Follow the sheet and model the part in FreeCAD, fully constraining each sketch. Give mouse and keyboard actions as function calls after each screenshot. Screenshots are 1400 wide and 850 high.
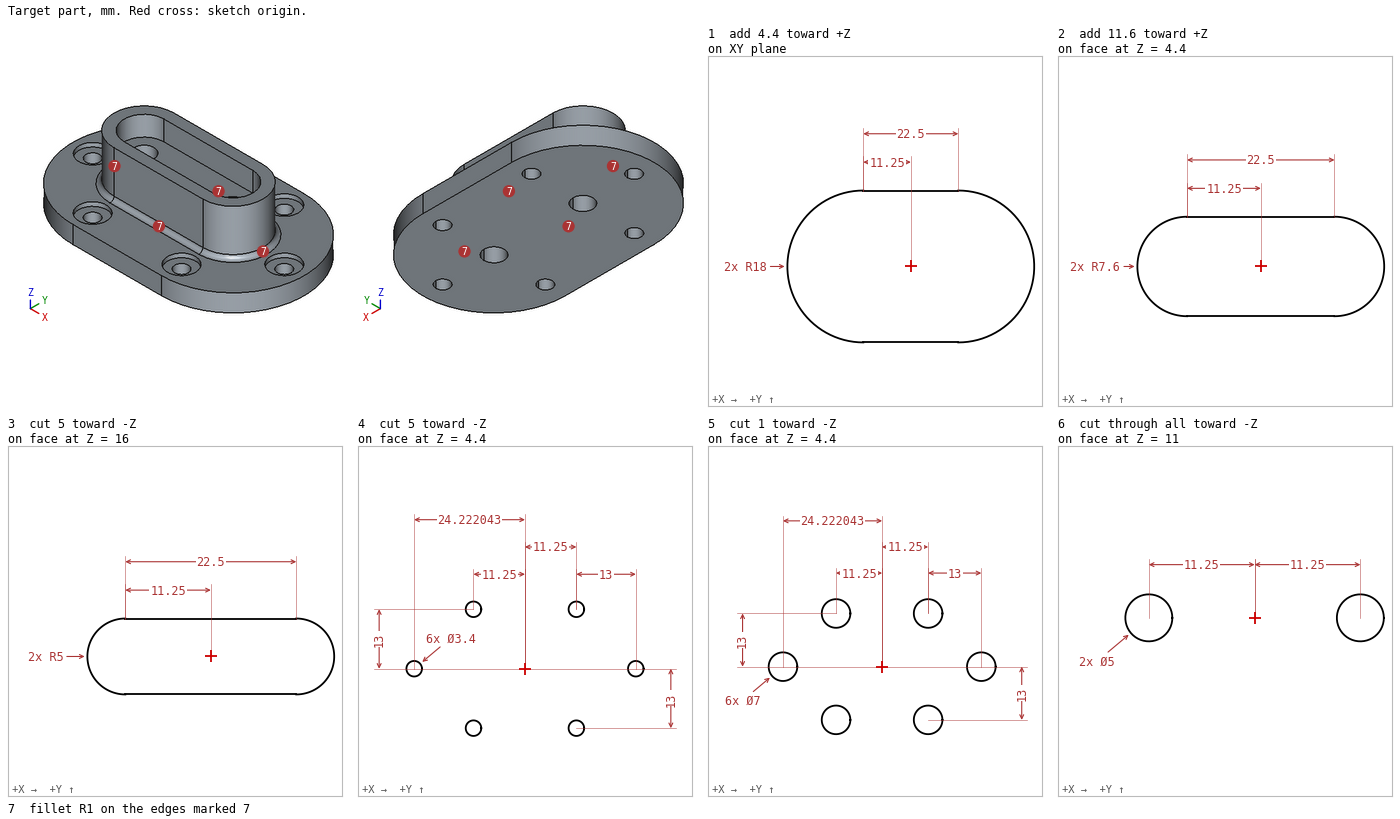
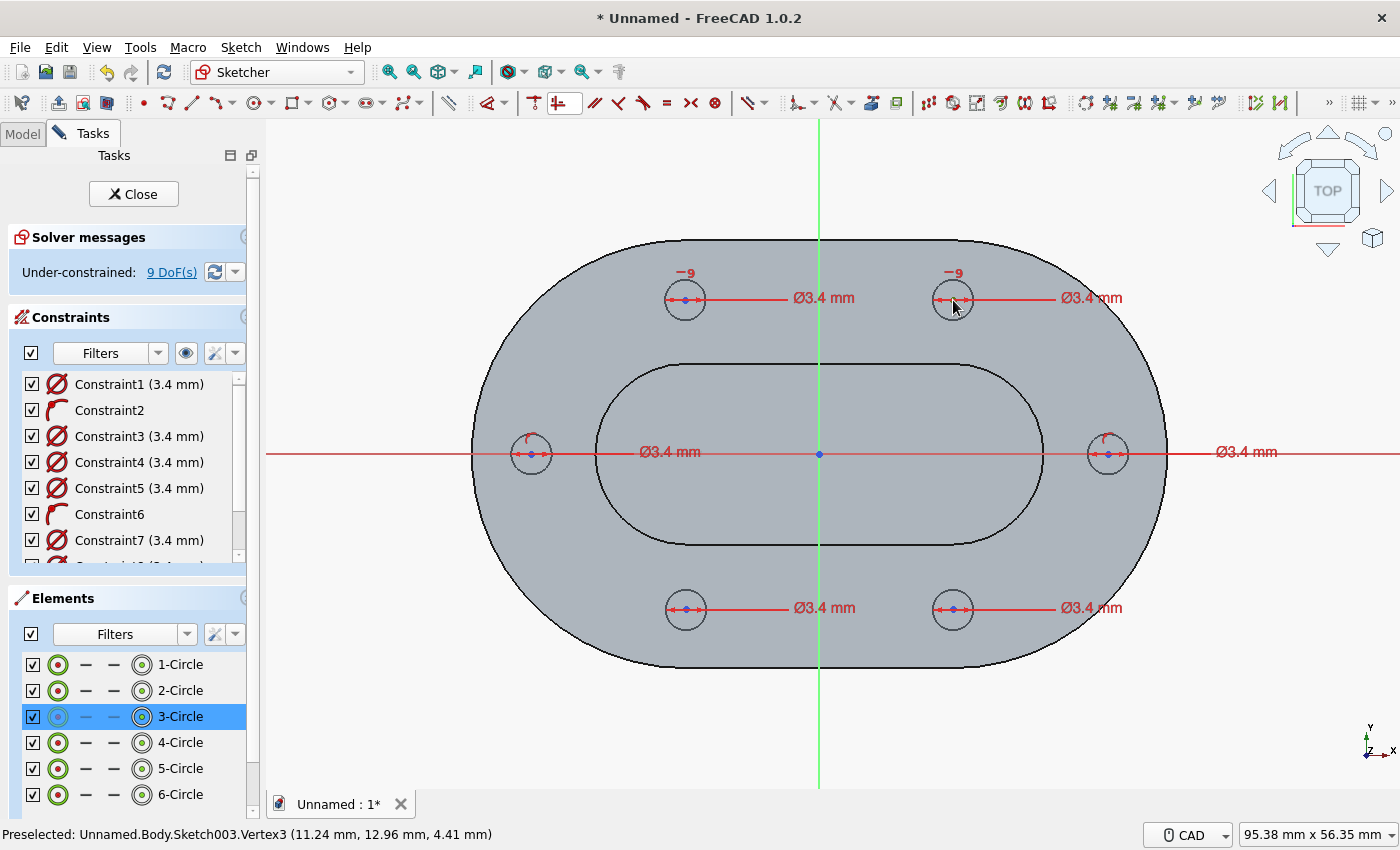
click(953, 610)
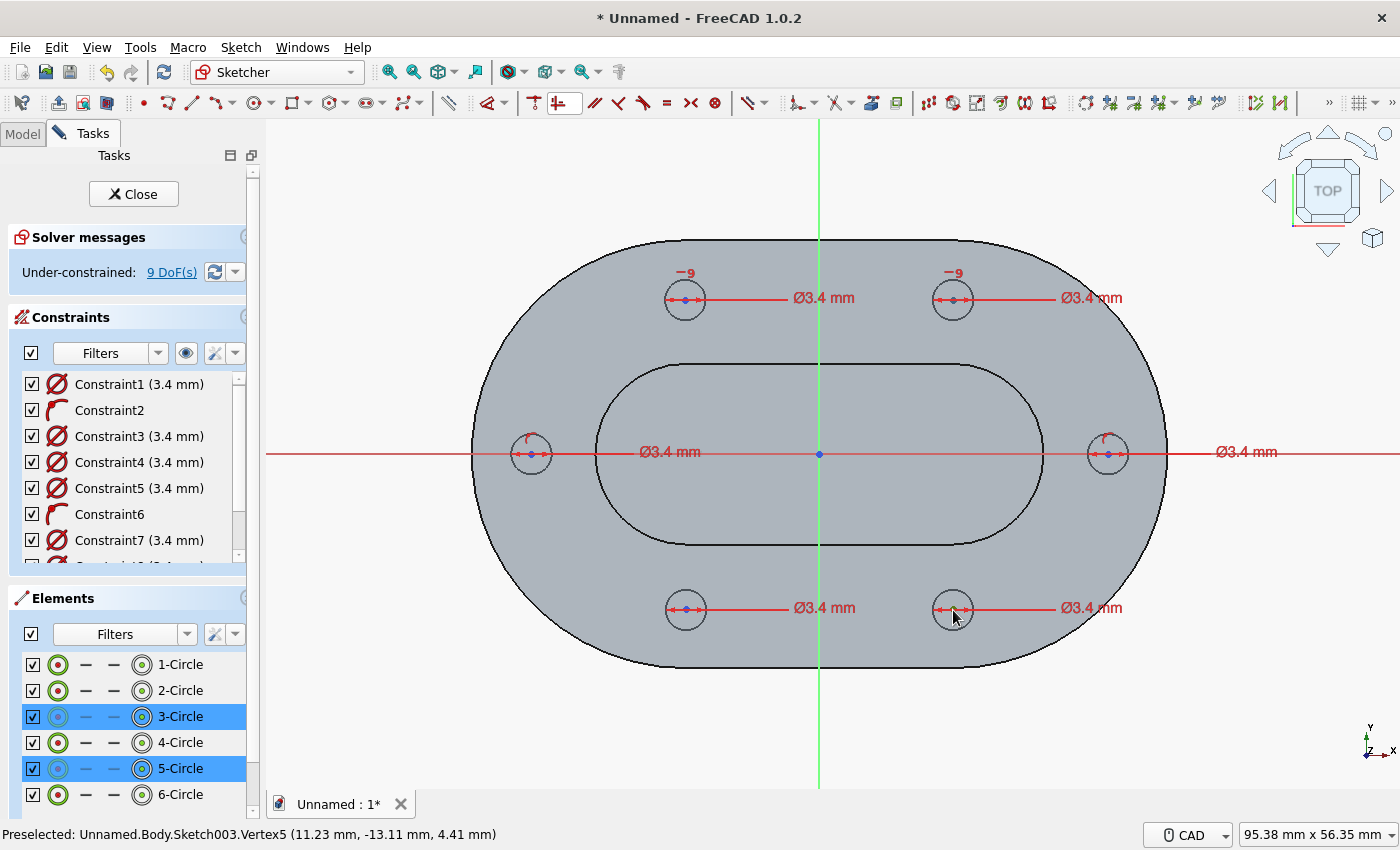
key(v)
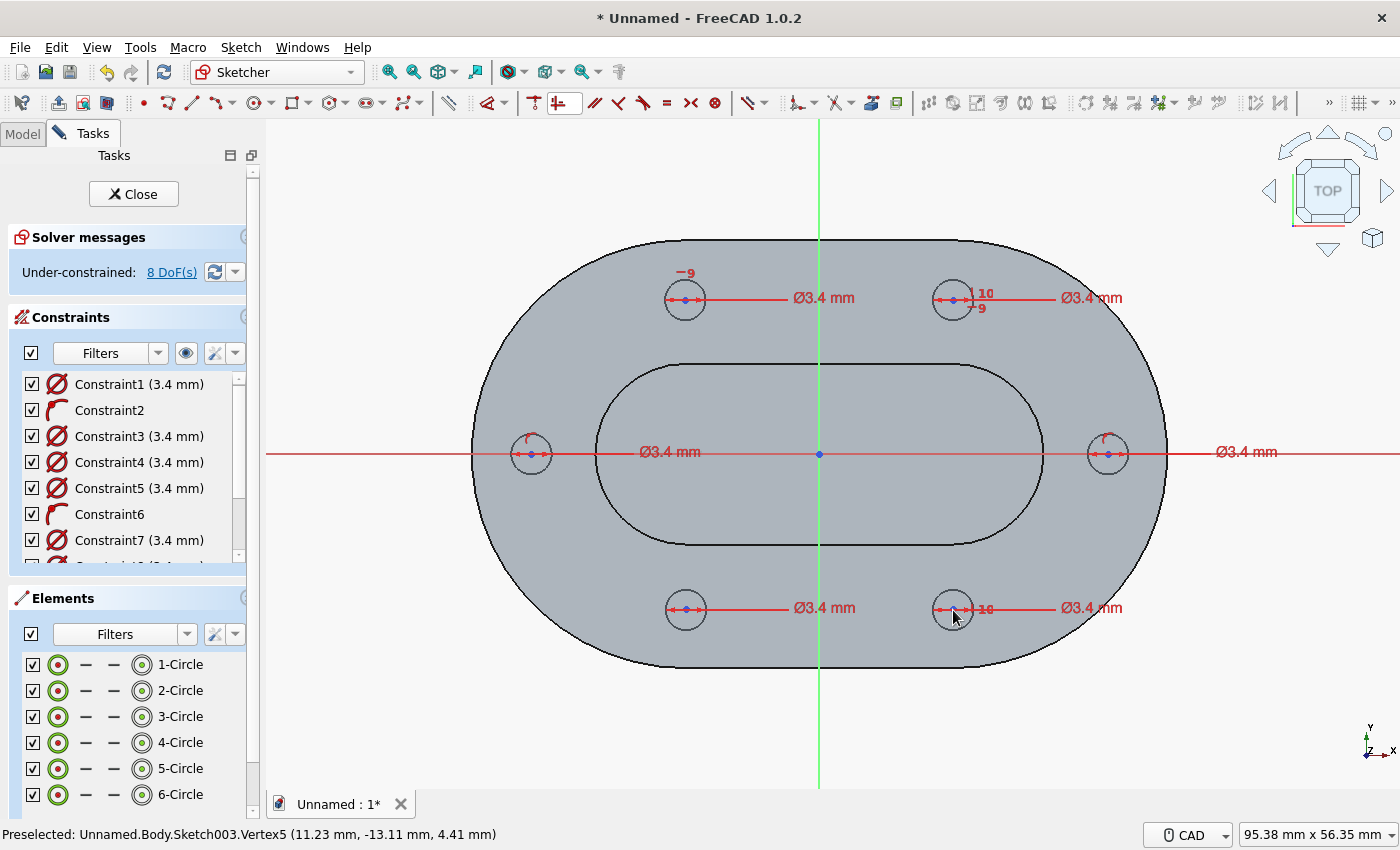
click(685, 300)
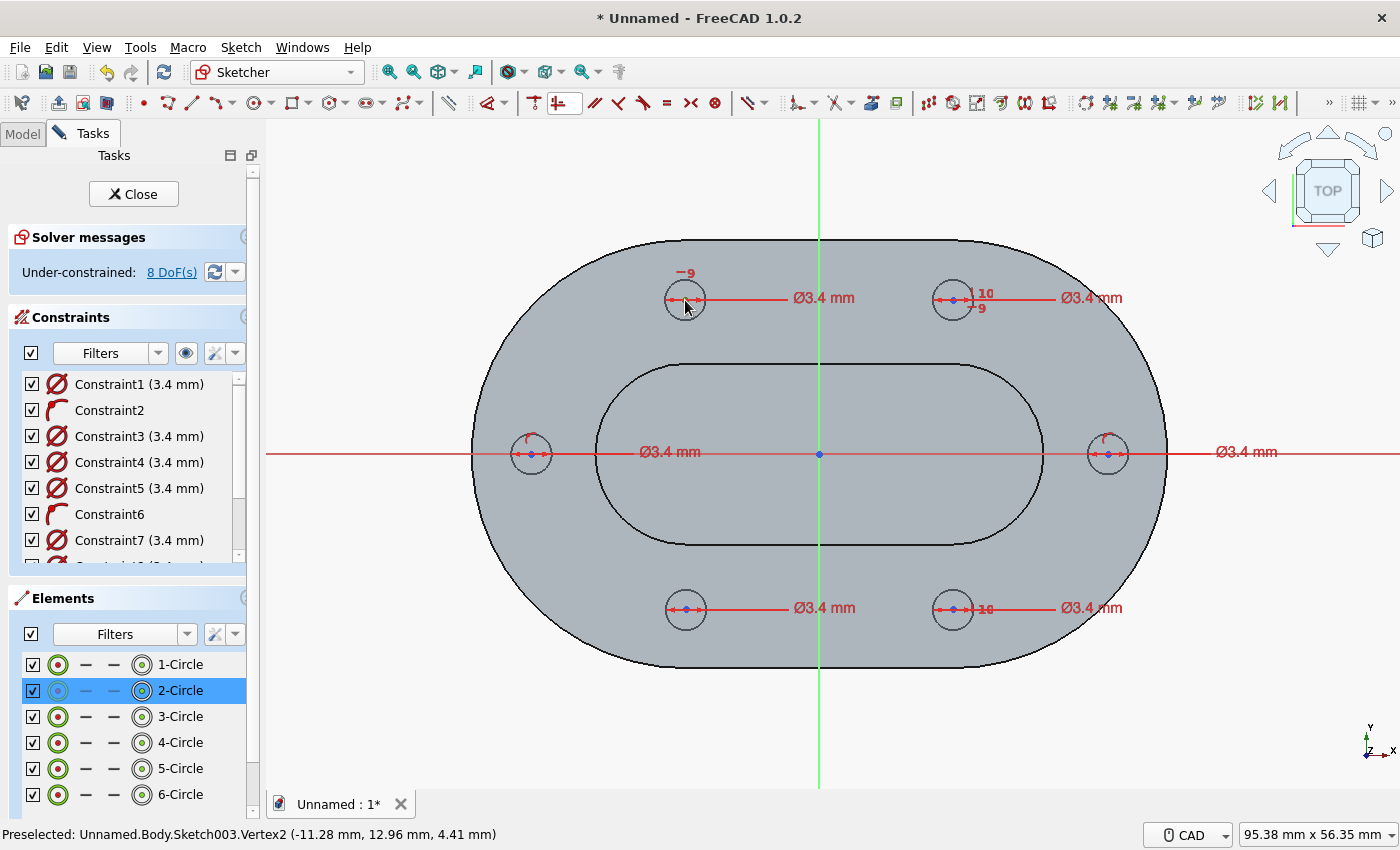
click(686, 610)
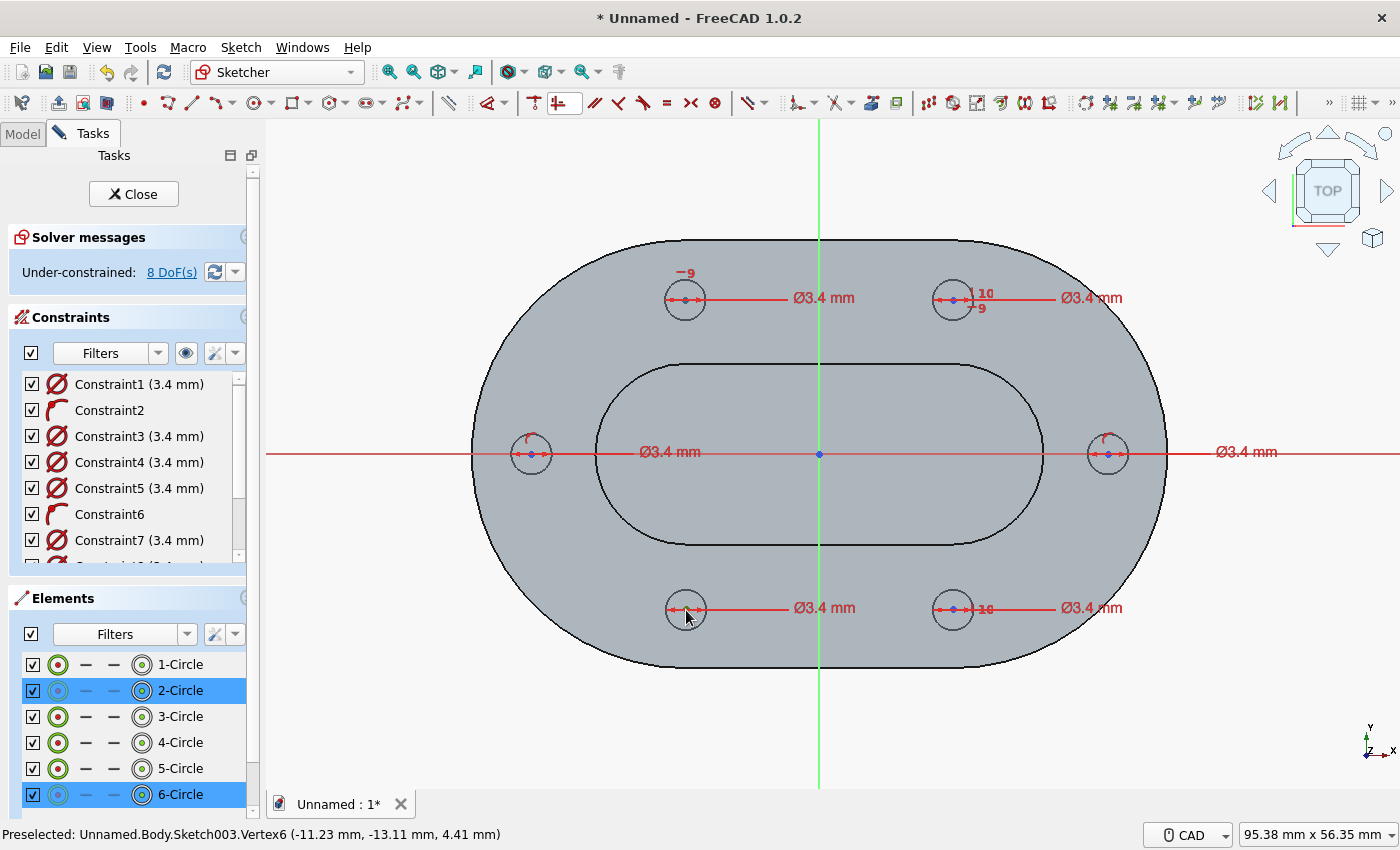
key(v)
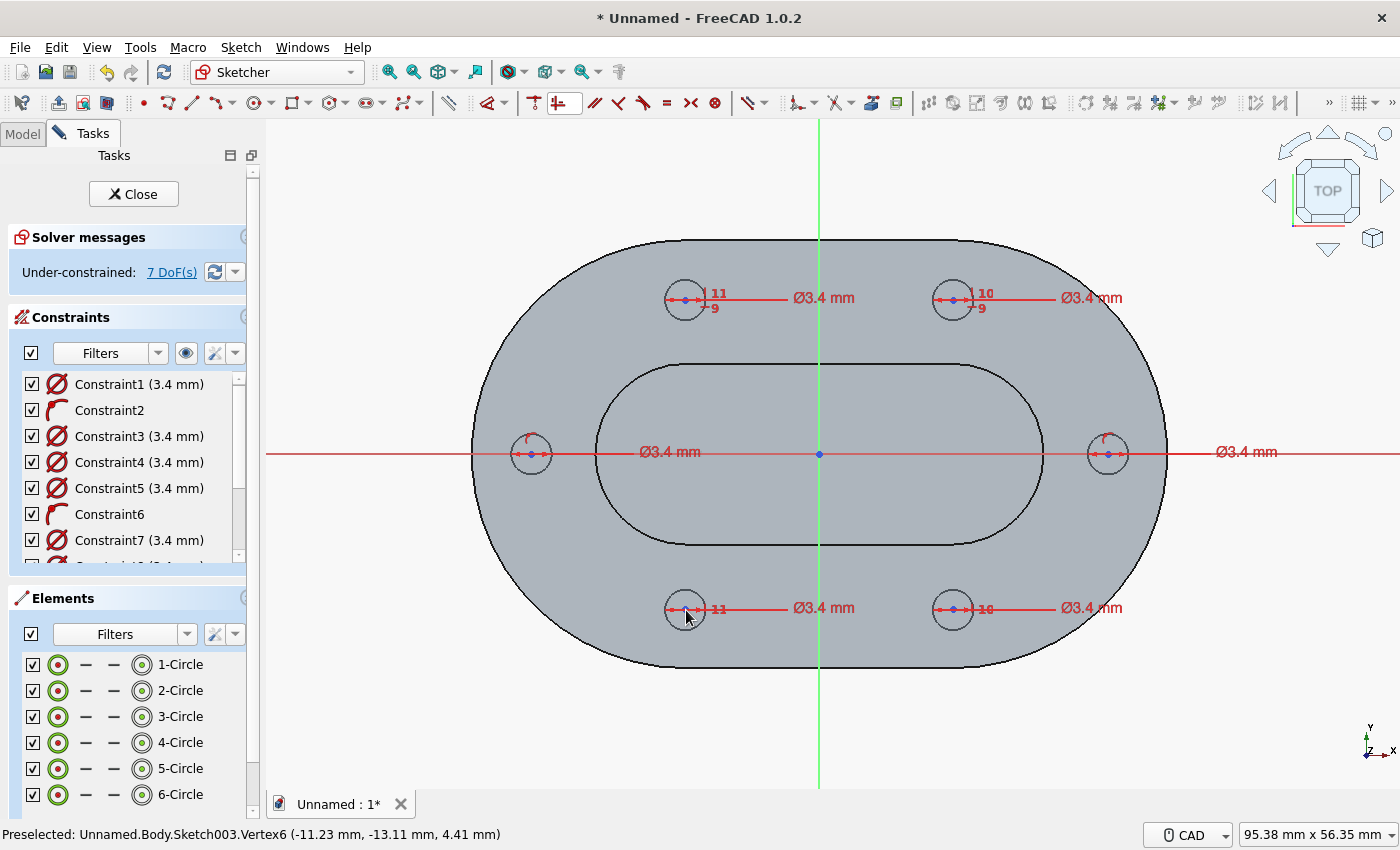
click(953, 610)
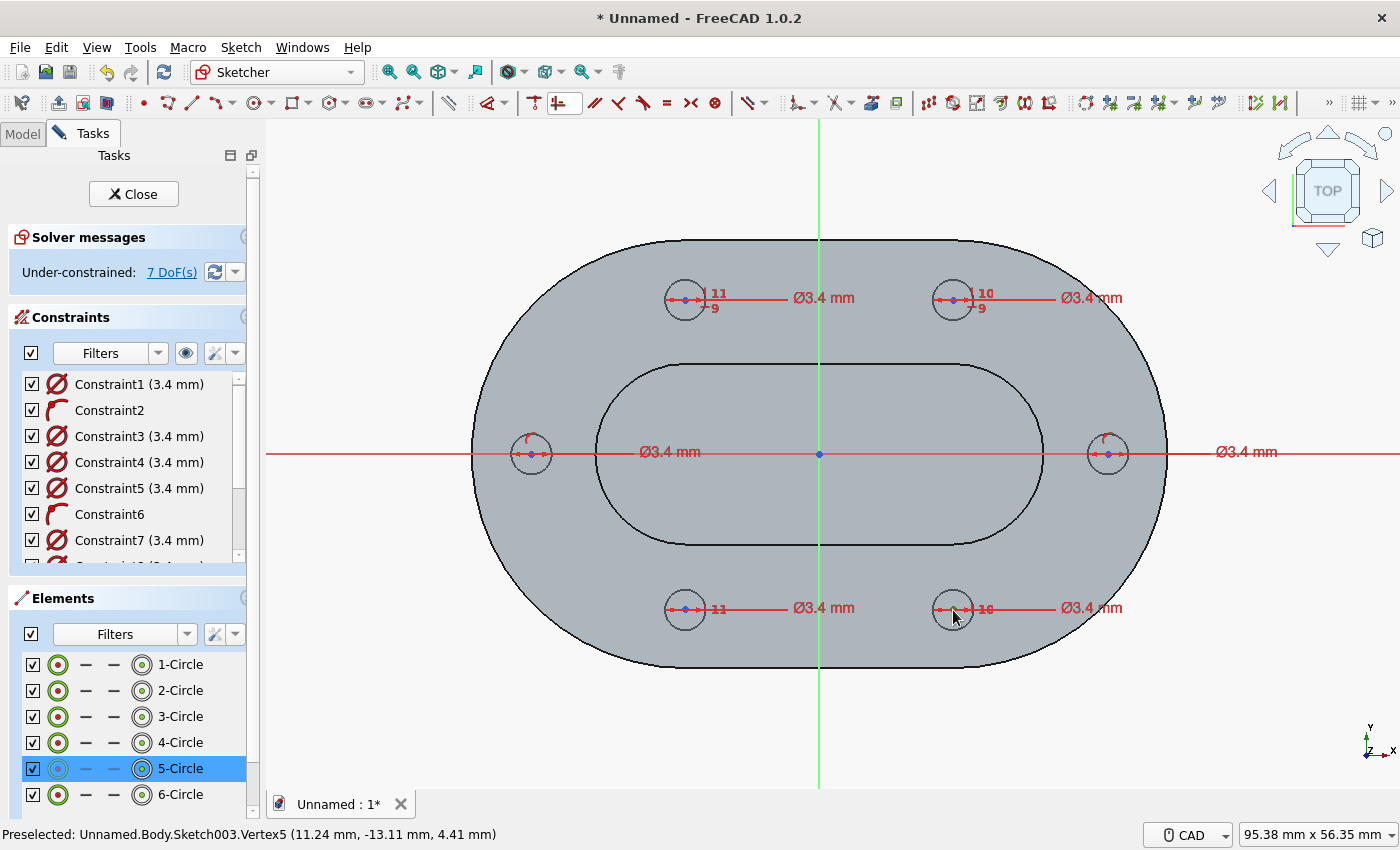
click(685, 610)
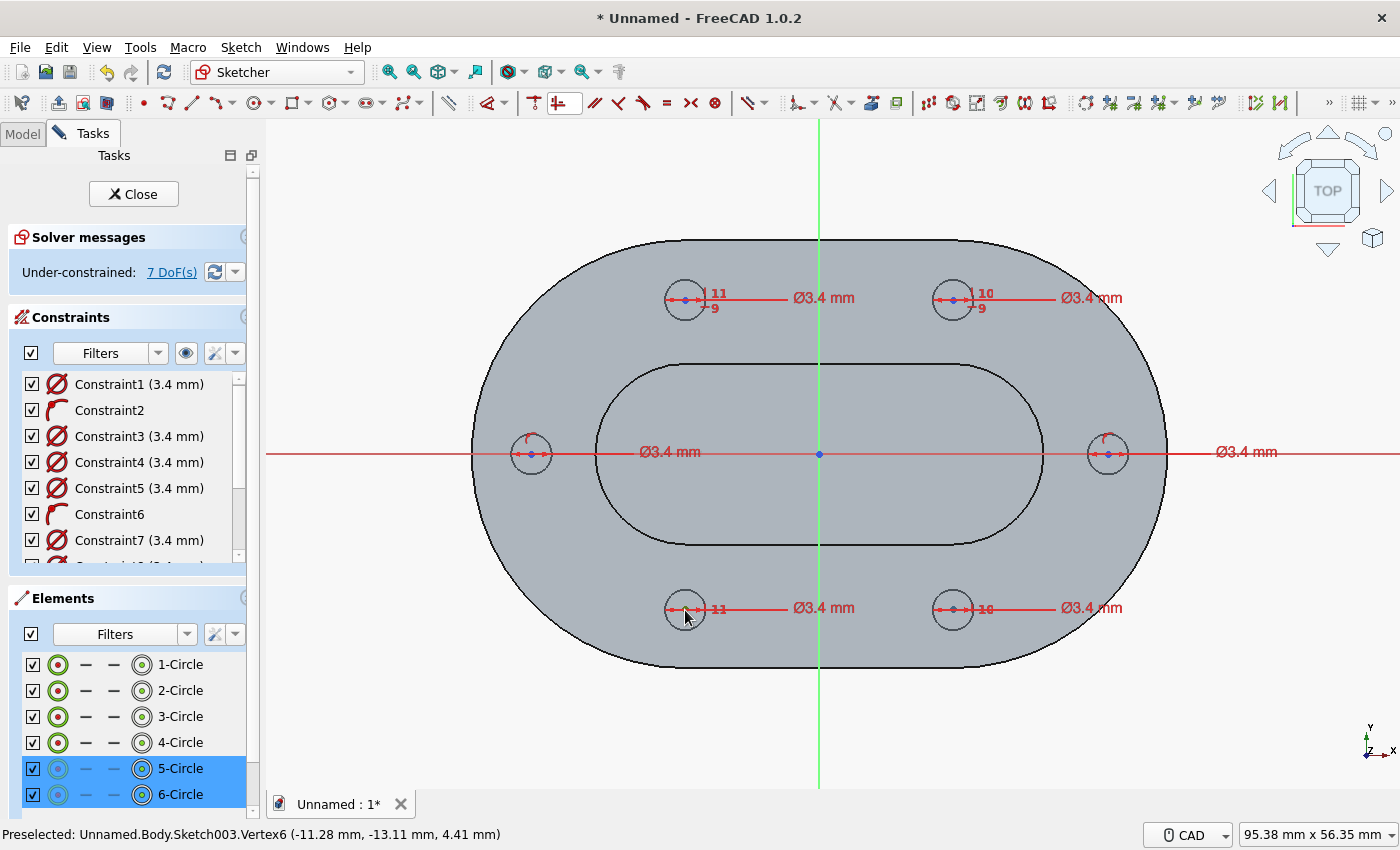
click(576, 104)